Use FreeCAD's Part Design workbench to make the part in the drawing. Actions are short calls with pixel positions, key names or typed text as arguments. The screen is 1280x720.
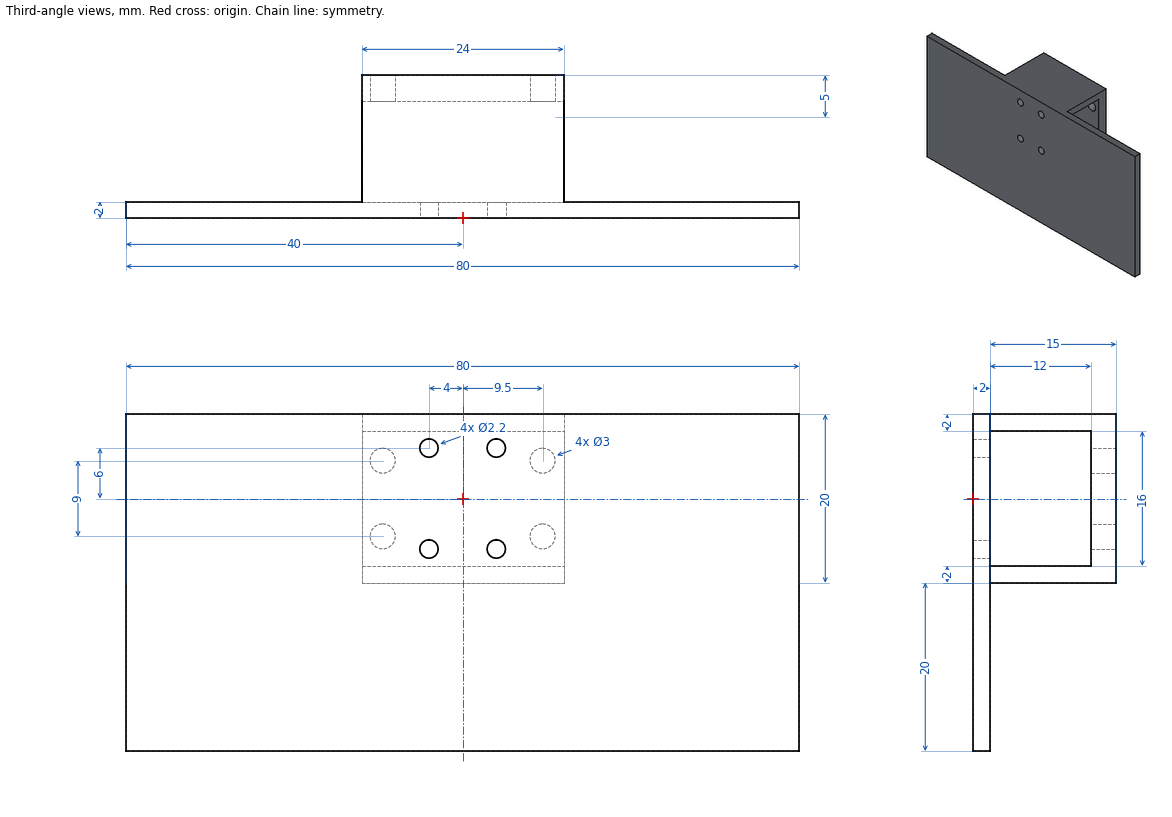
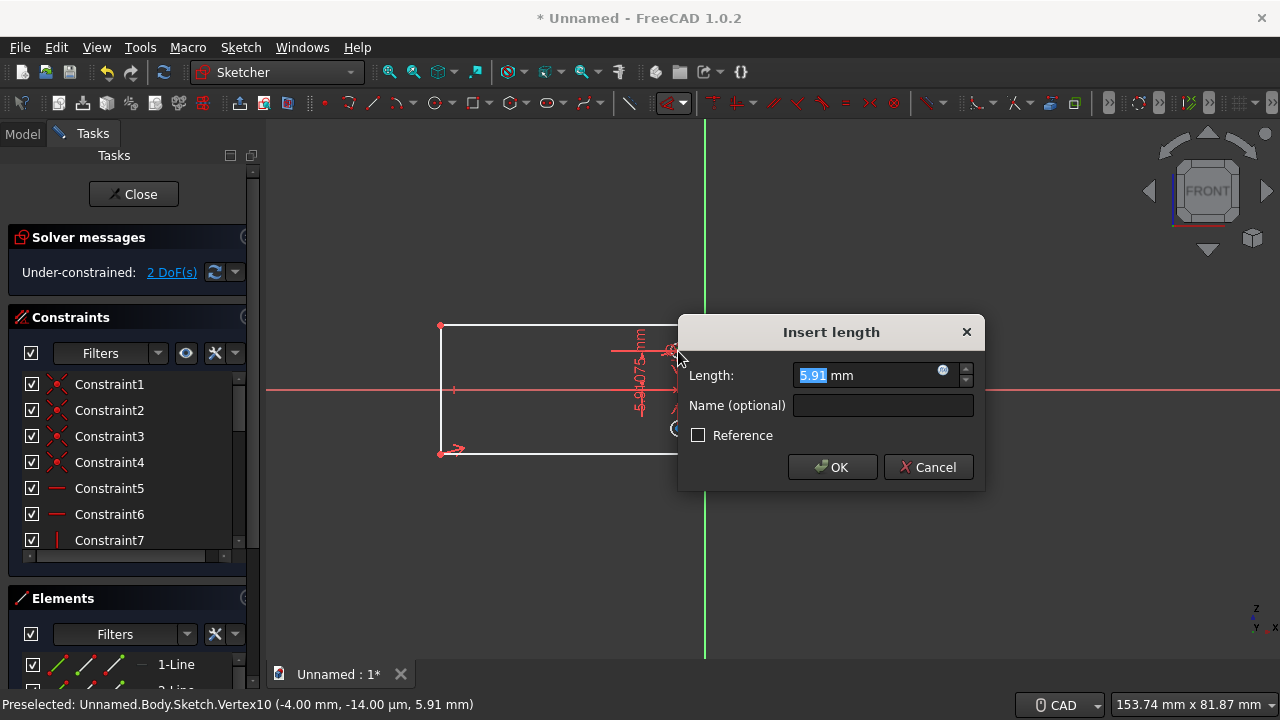
text(6)
key(Return)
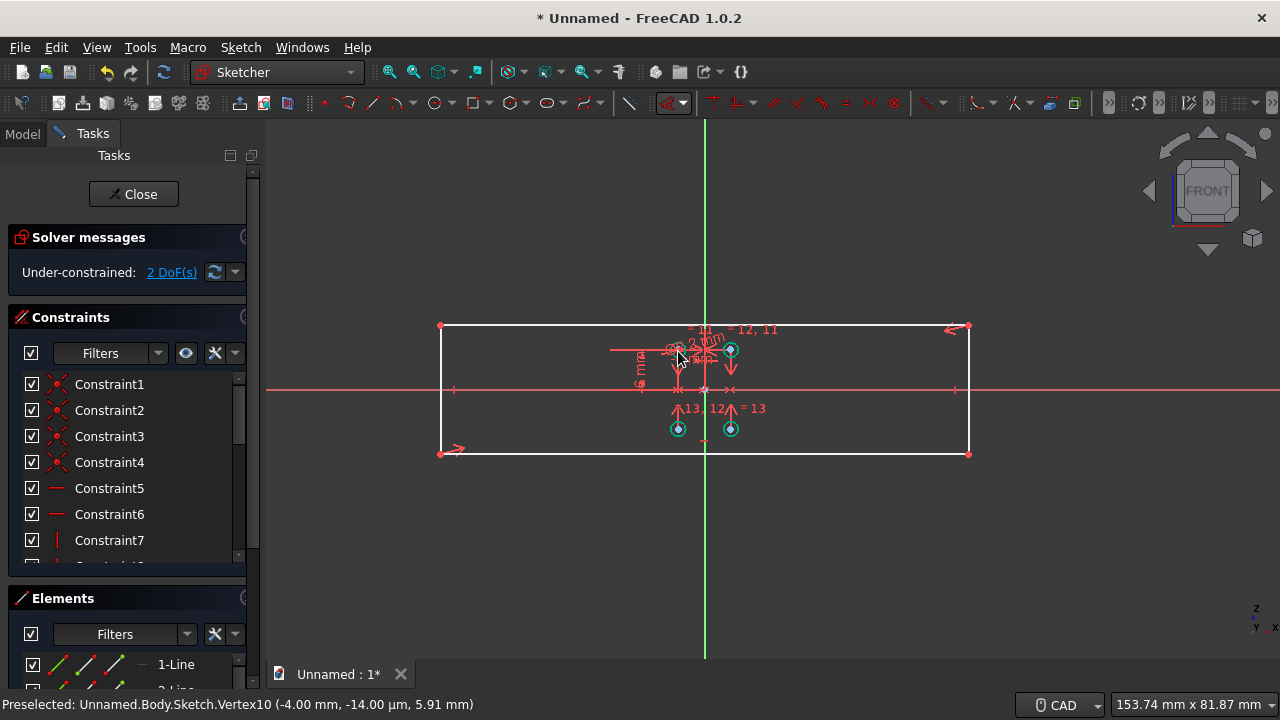
click(599, 454)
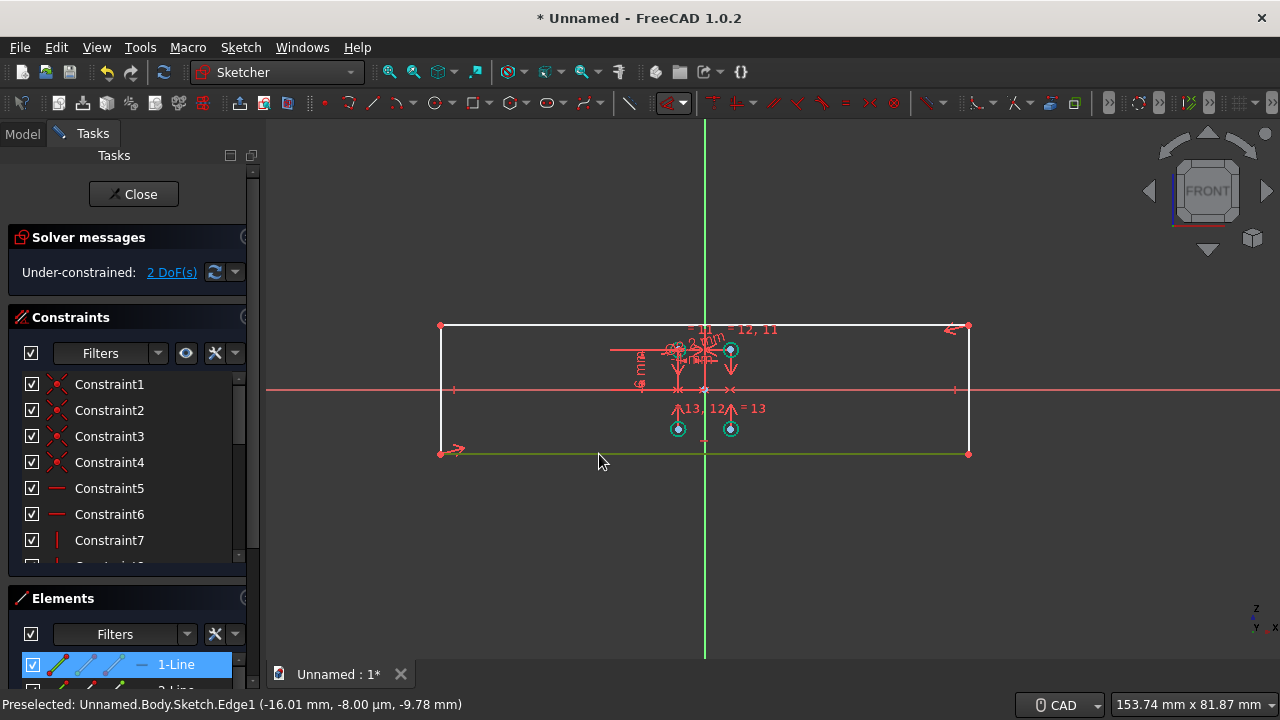
click(686, 104)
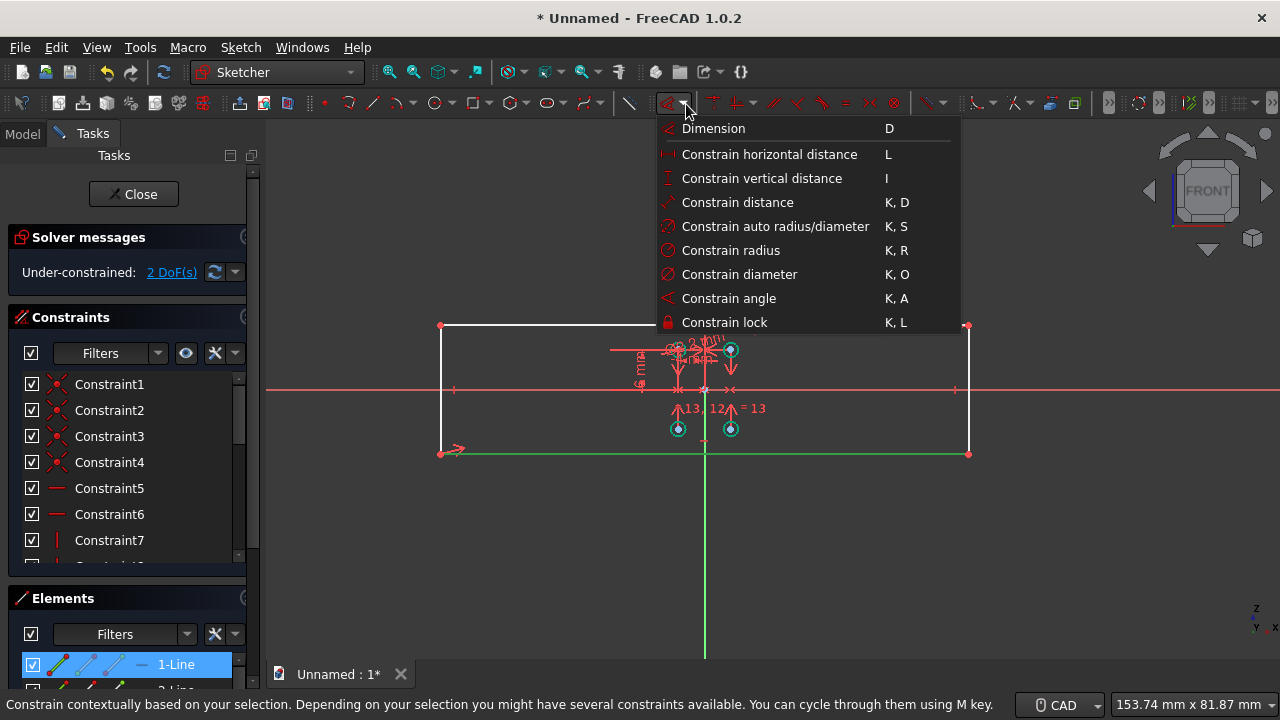
click(809, 154)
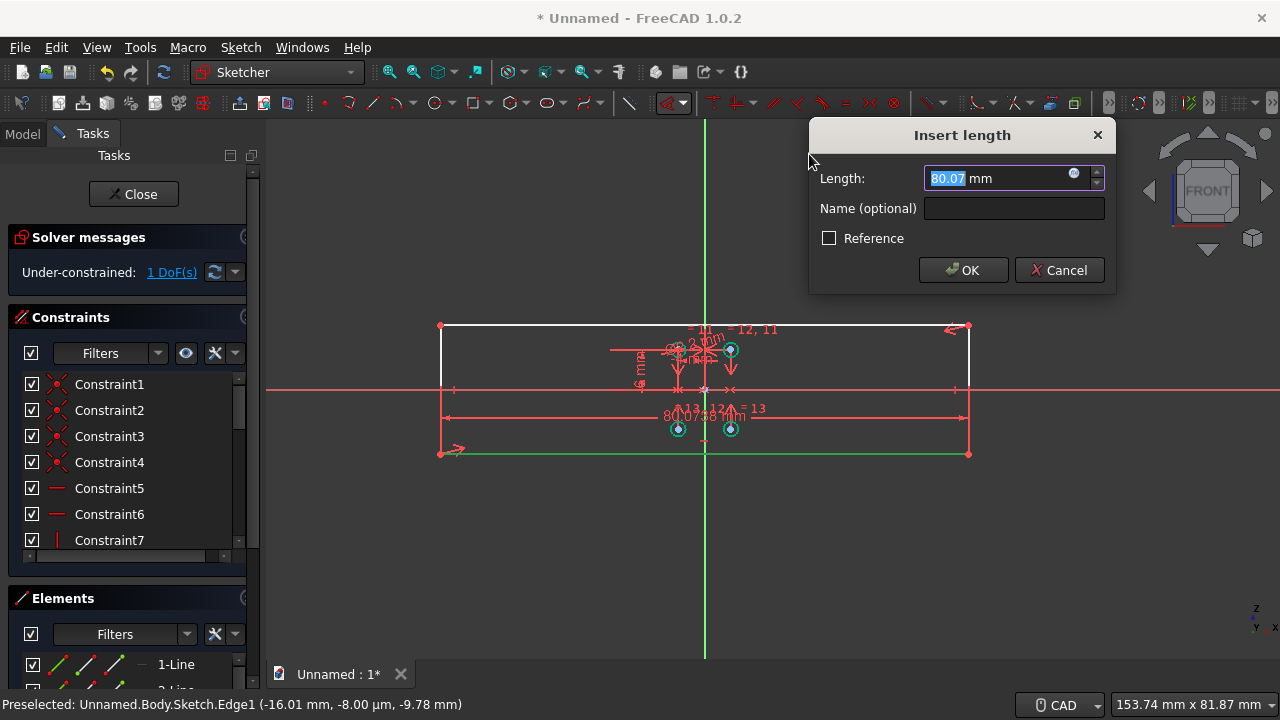
text(80)
key(Return)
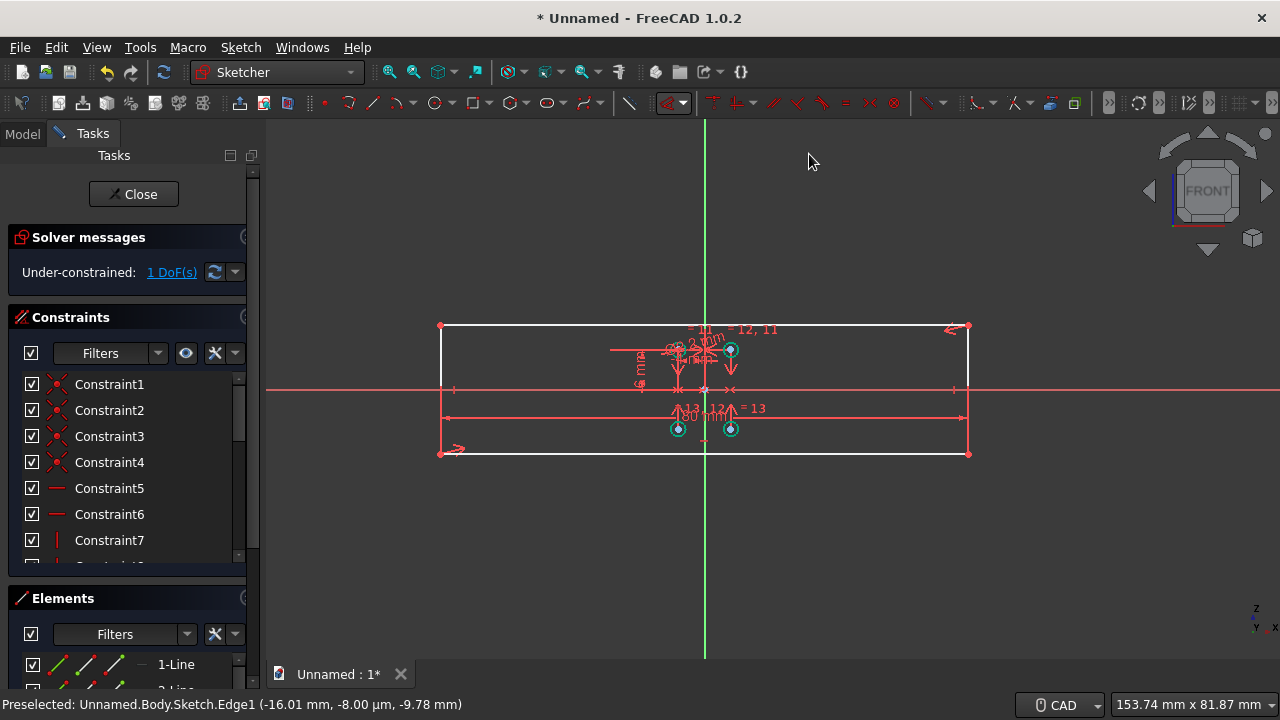
click(968, 415)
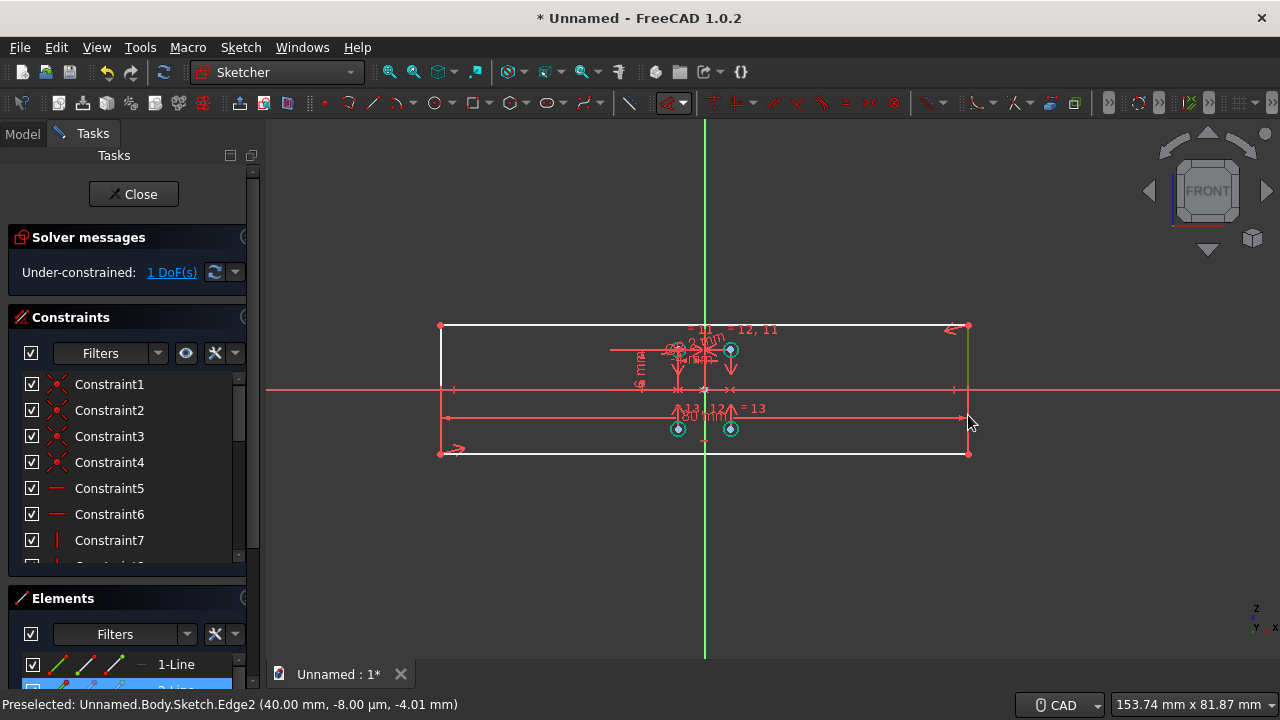
key(i)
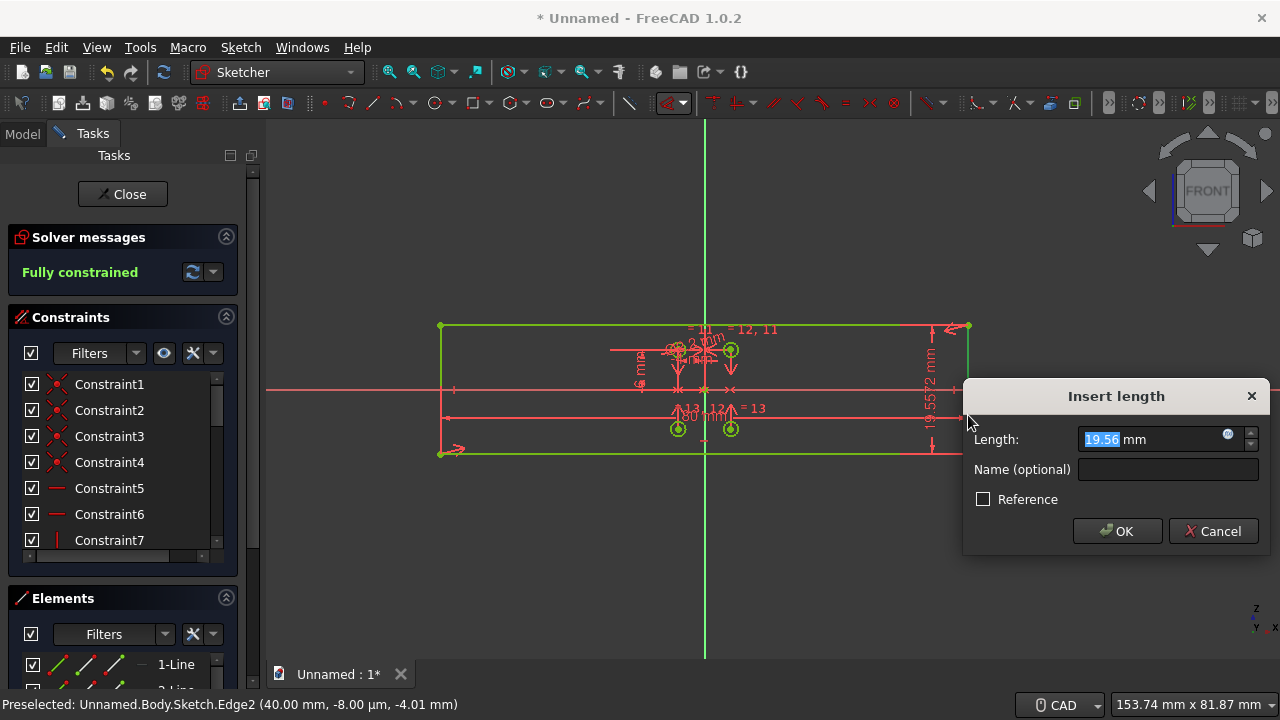
text(20)
key(Return)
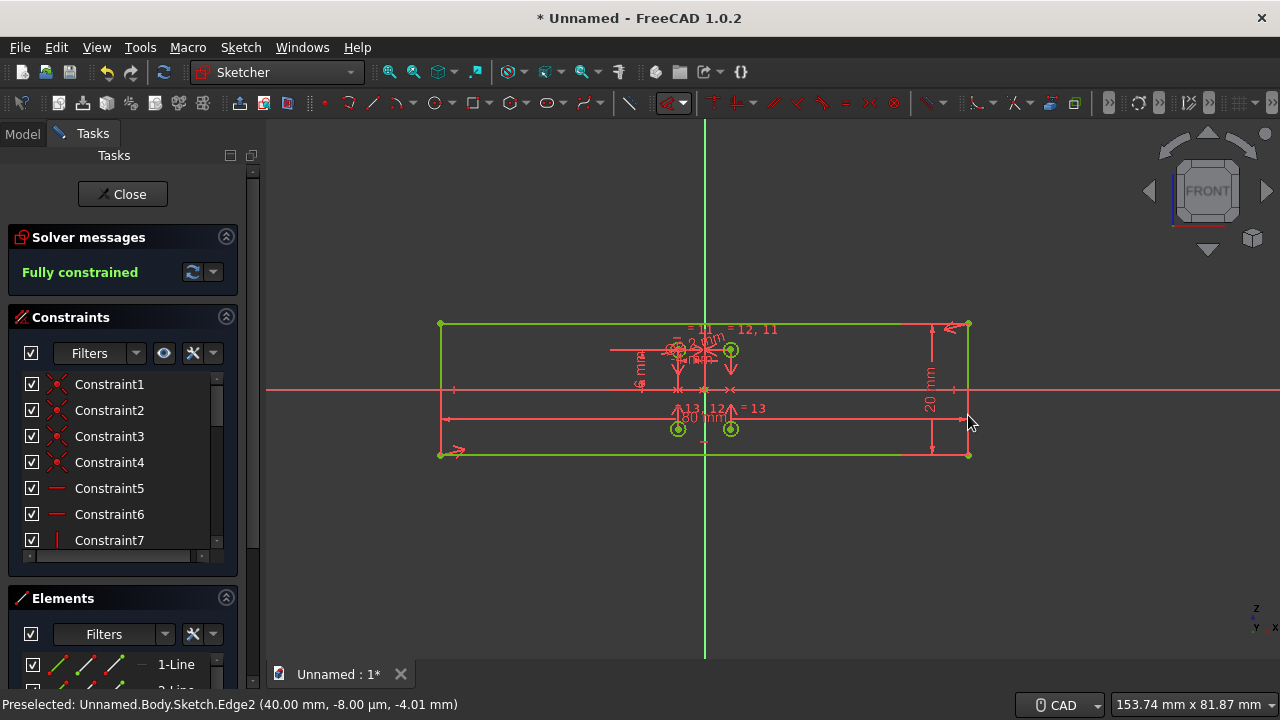
click(123, 194)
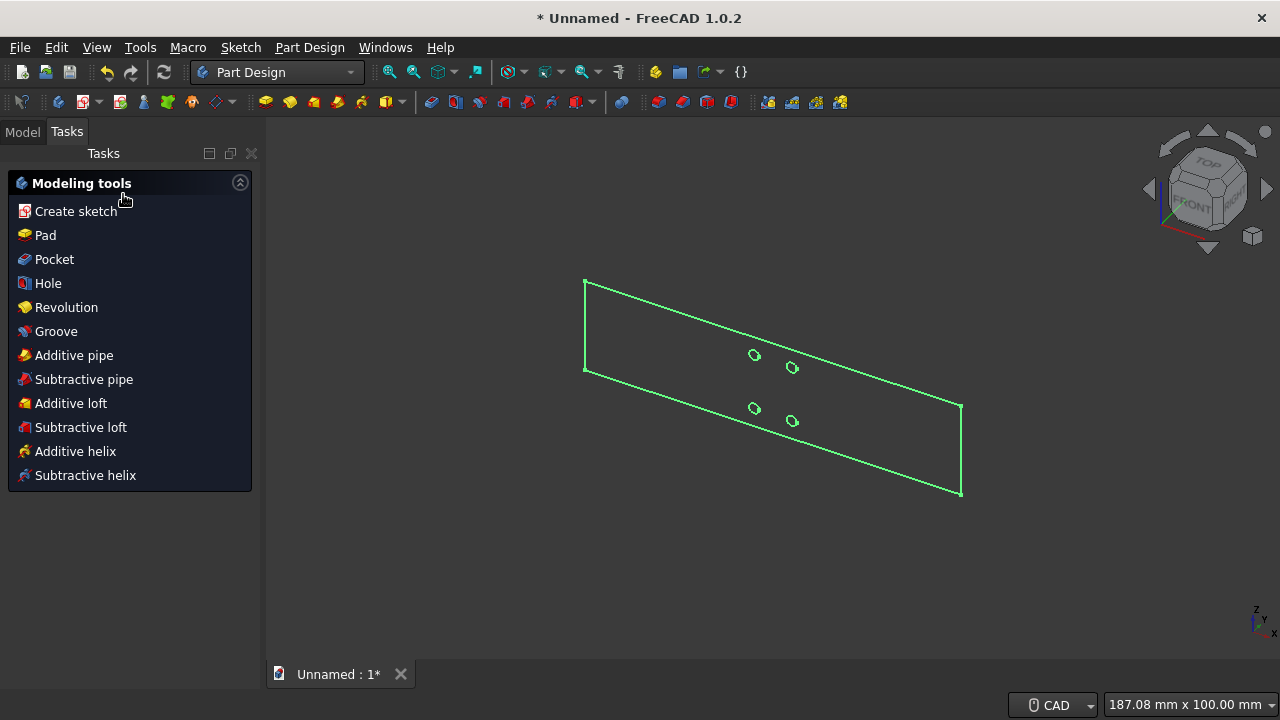
click(266, 102)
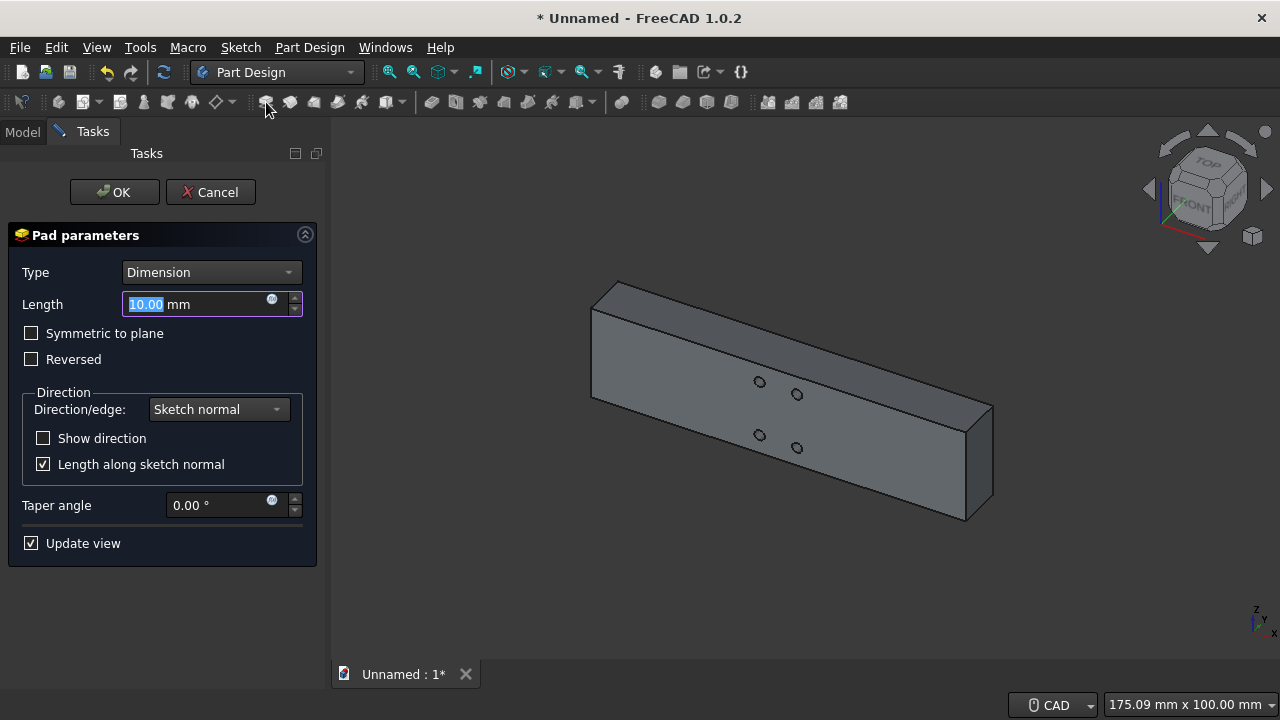
text(2)
key(Tab)